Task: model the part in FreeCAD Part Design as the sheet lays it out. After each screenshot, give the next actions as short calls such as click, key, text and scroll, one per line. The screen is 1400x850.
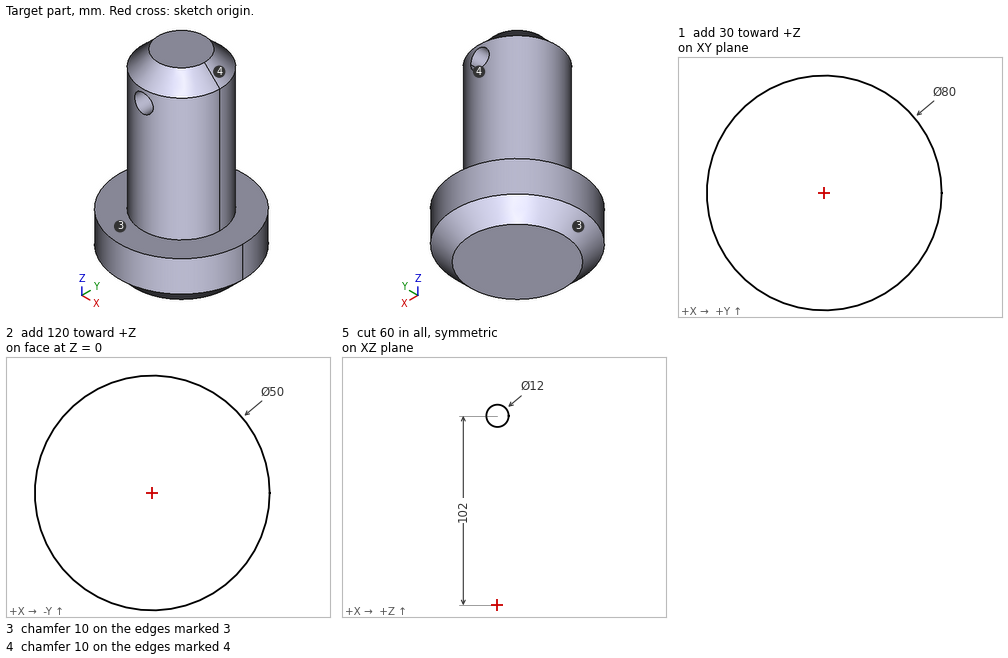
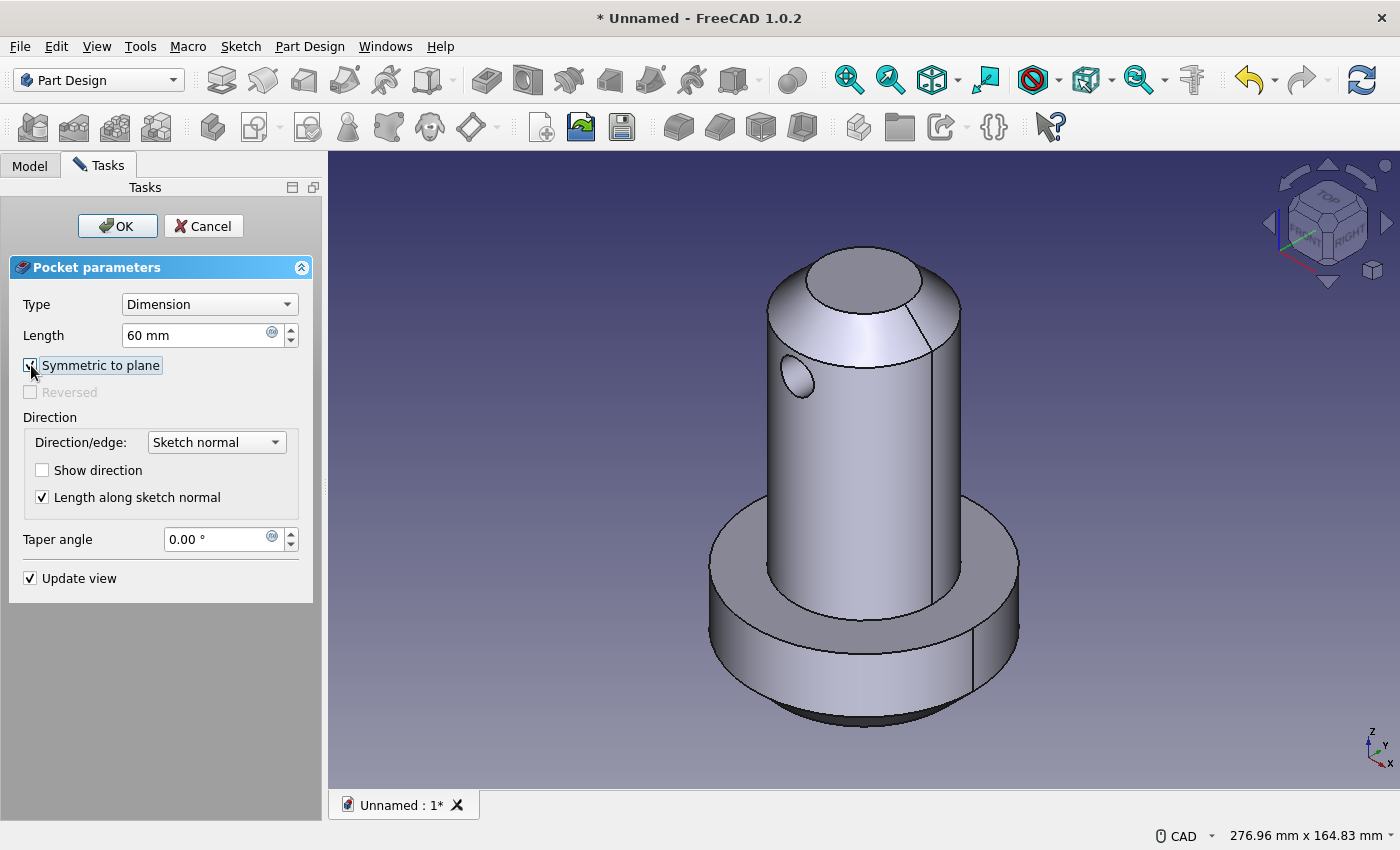
click(118, 226)